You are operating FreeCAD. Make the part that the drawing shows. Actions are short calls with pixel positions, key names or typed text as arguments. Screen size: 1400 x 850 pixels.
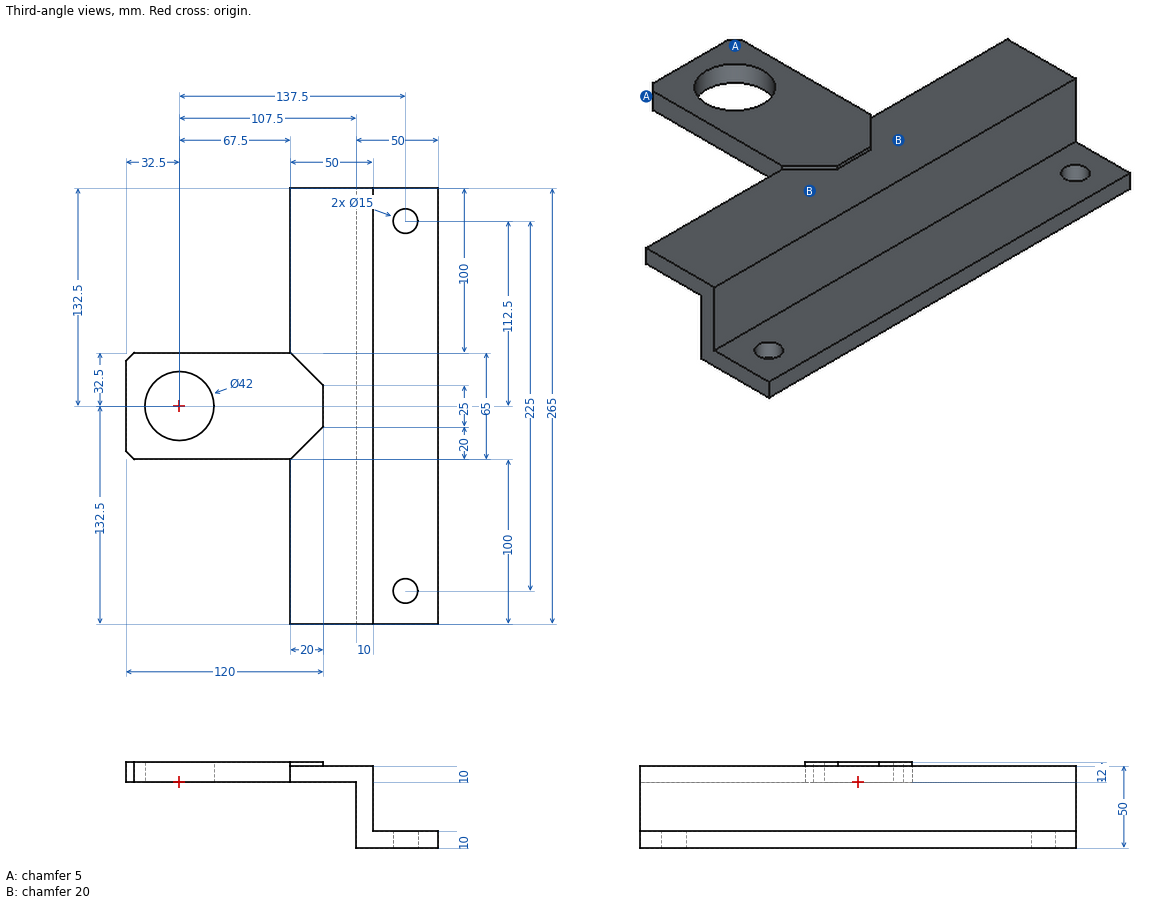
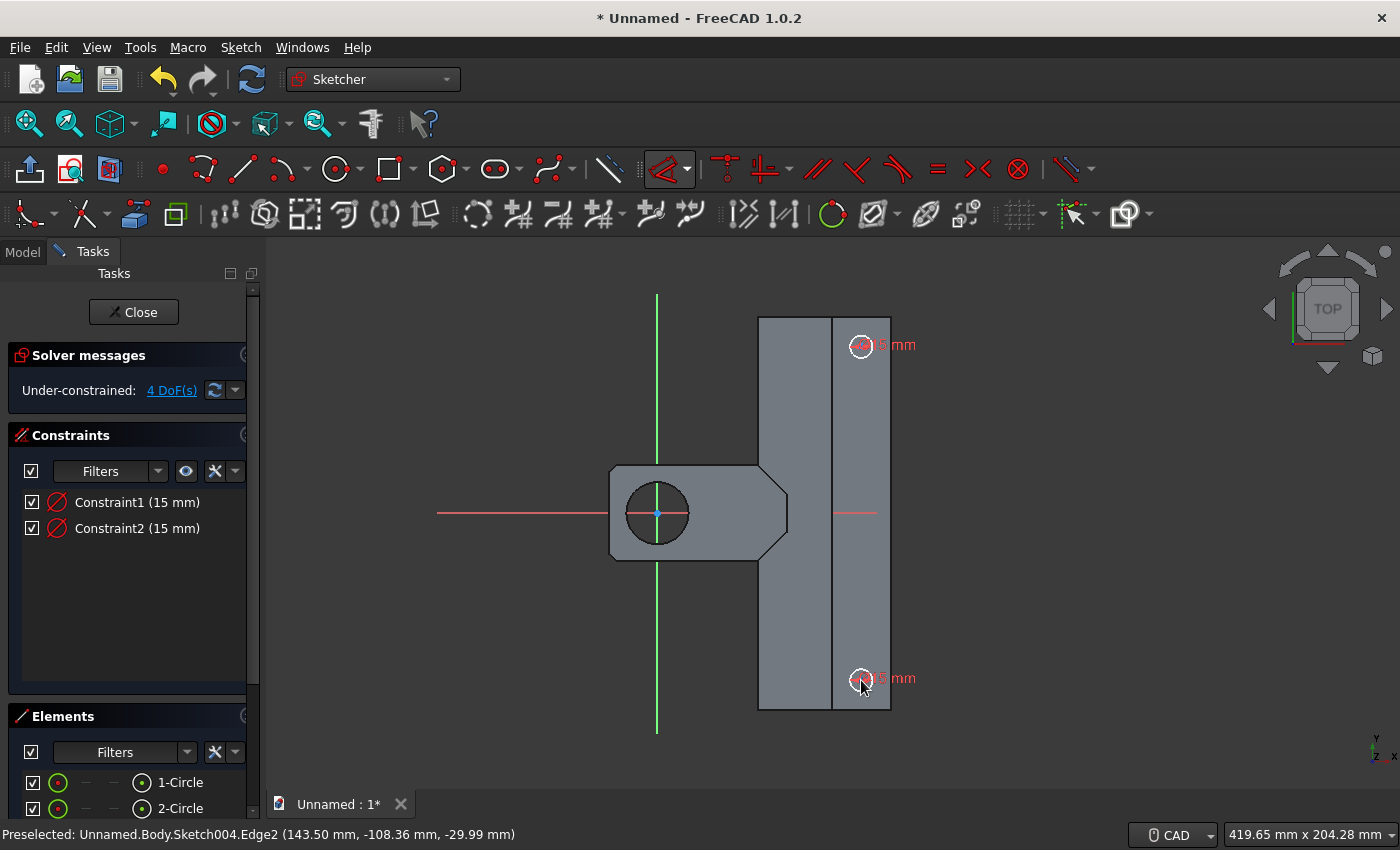
click(861, 347)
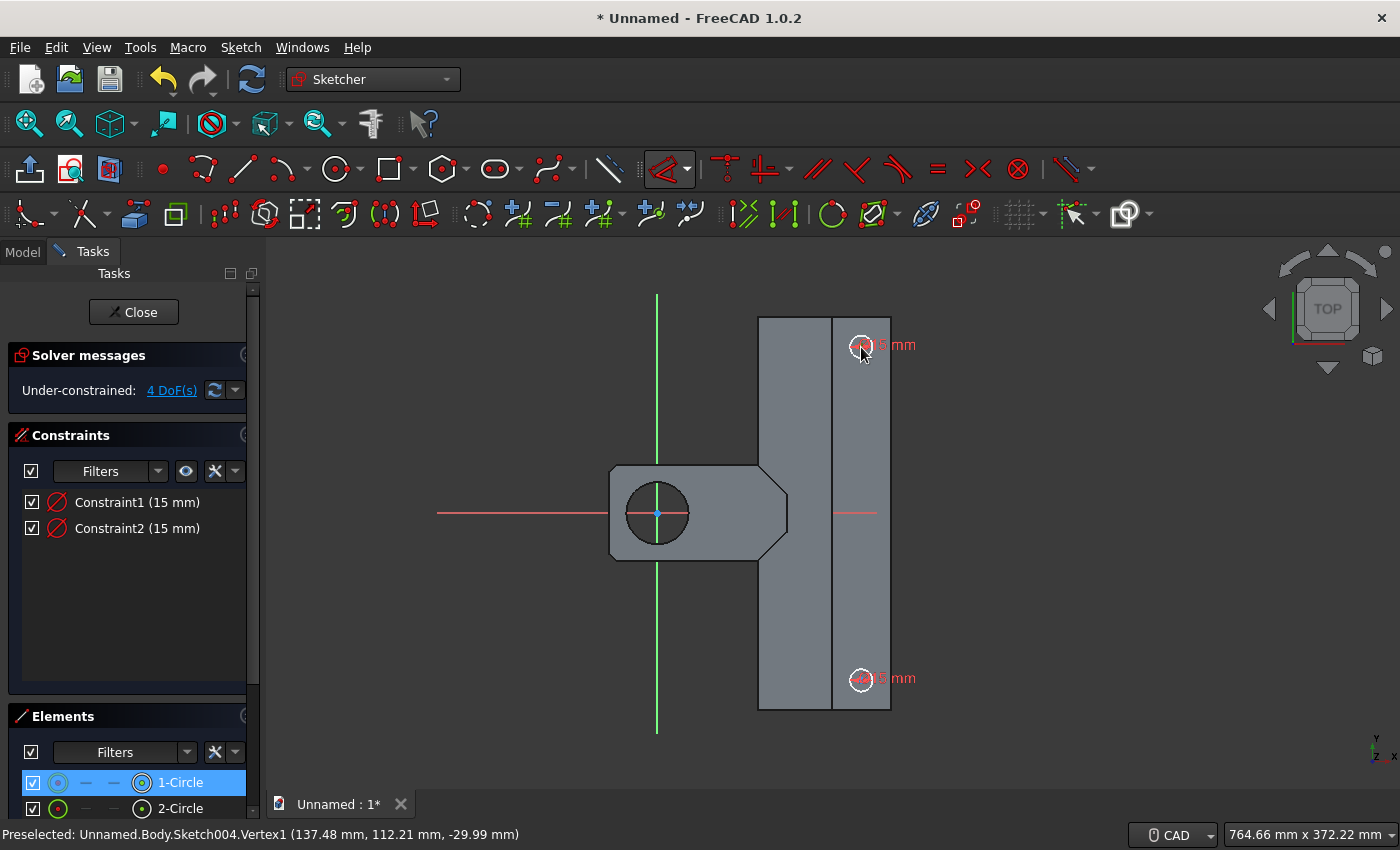
click(861, 680)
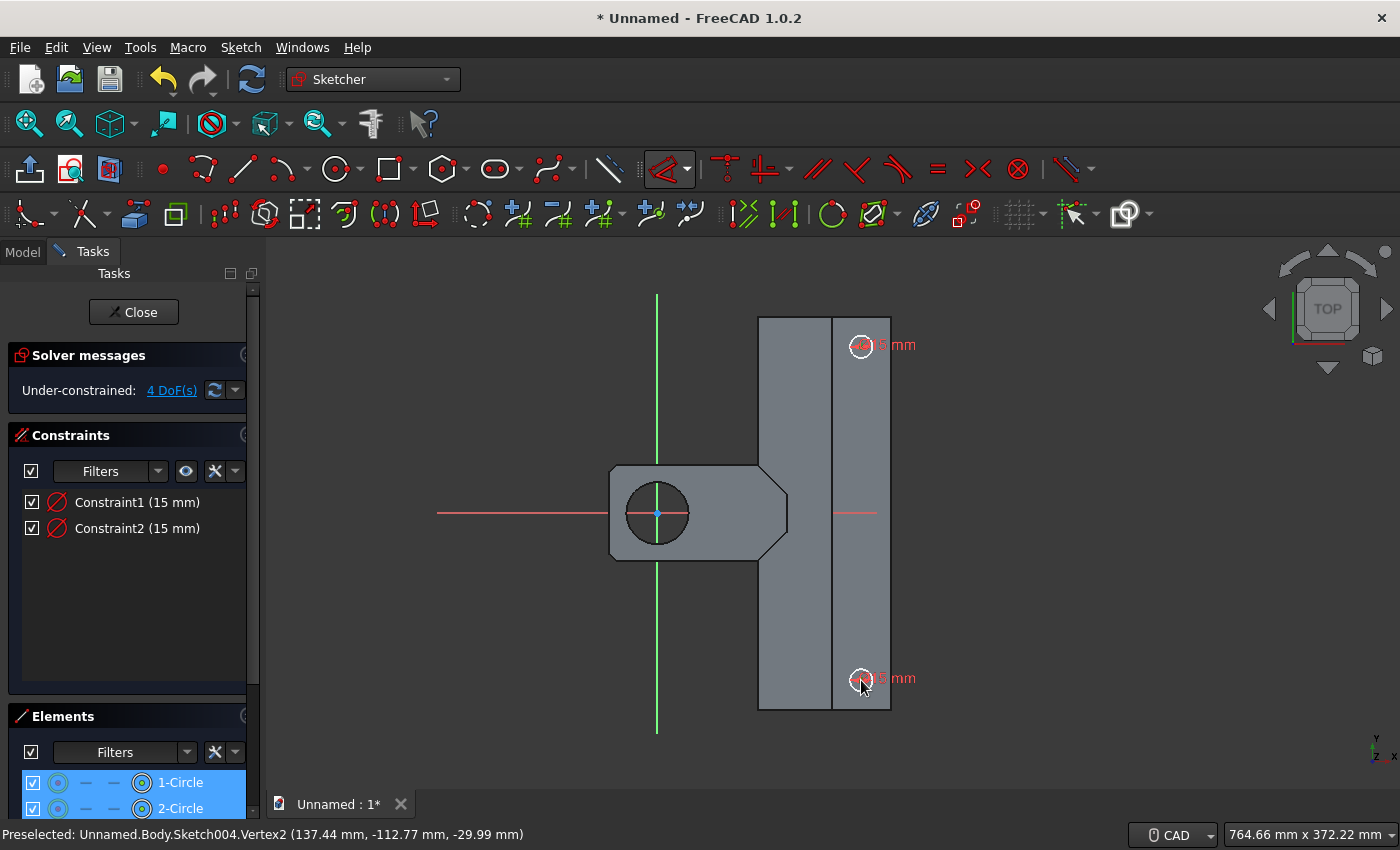
click(792, 170)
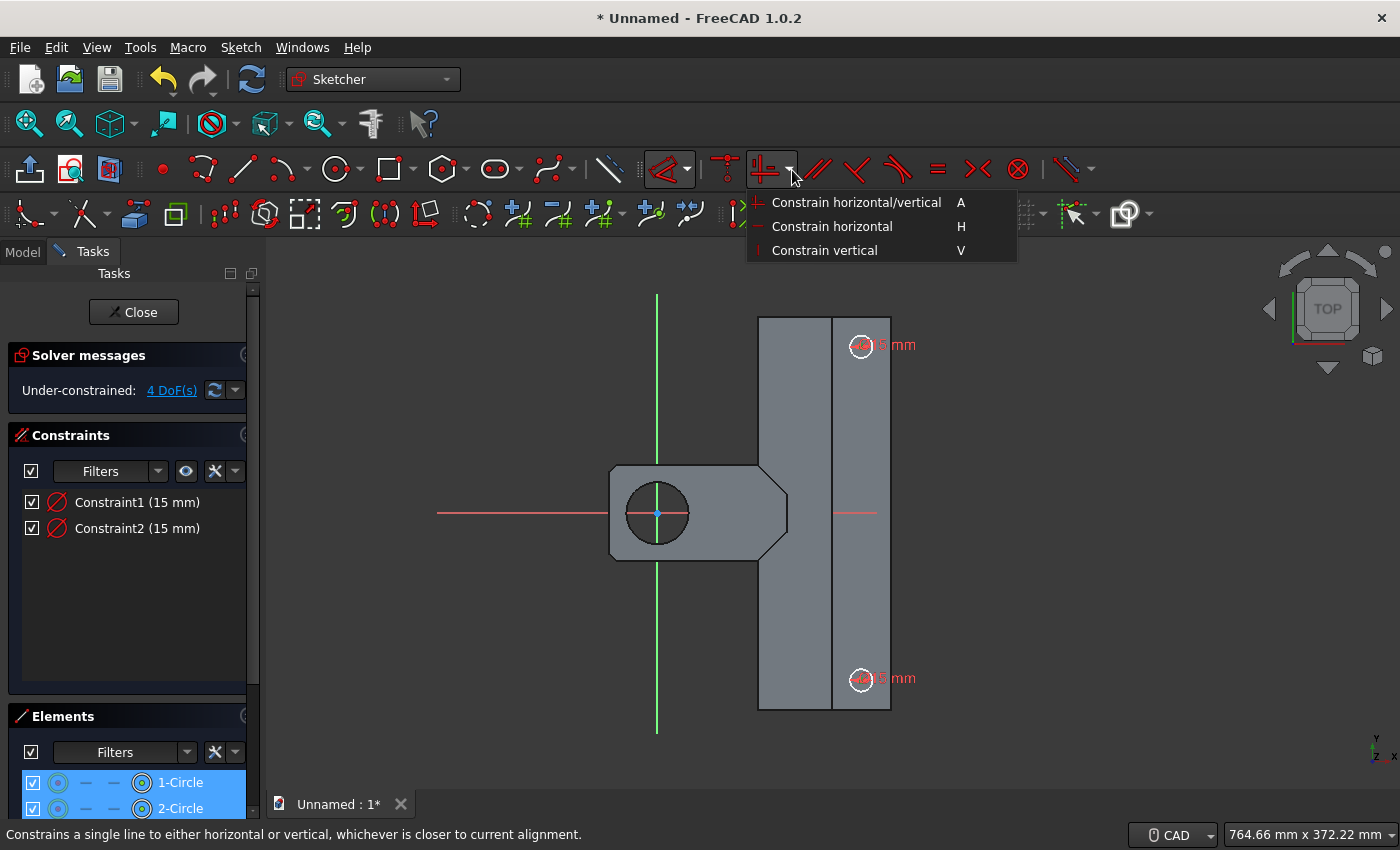
click(882, 250)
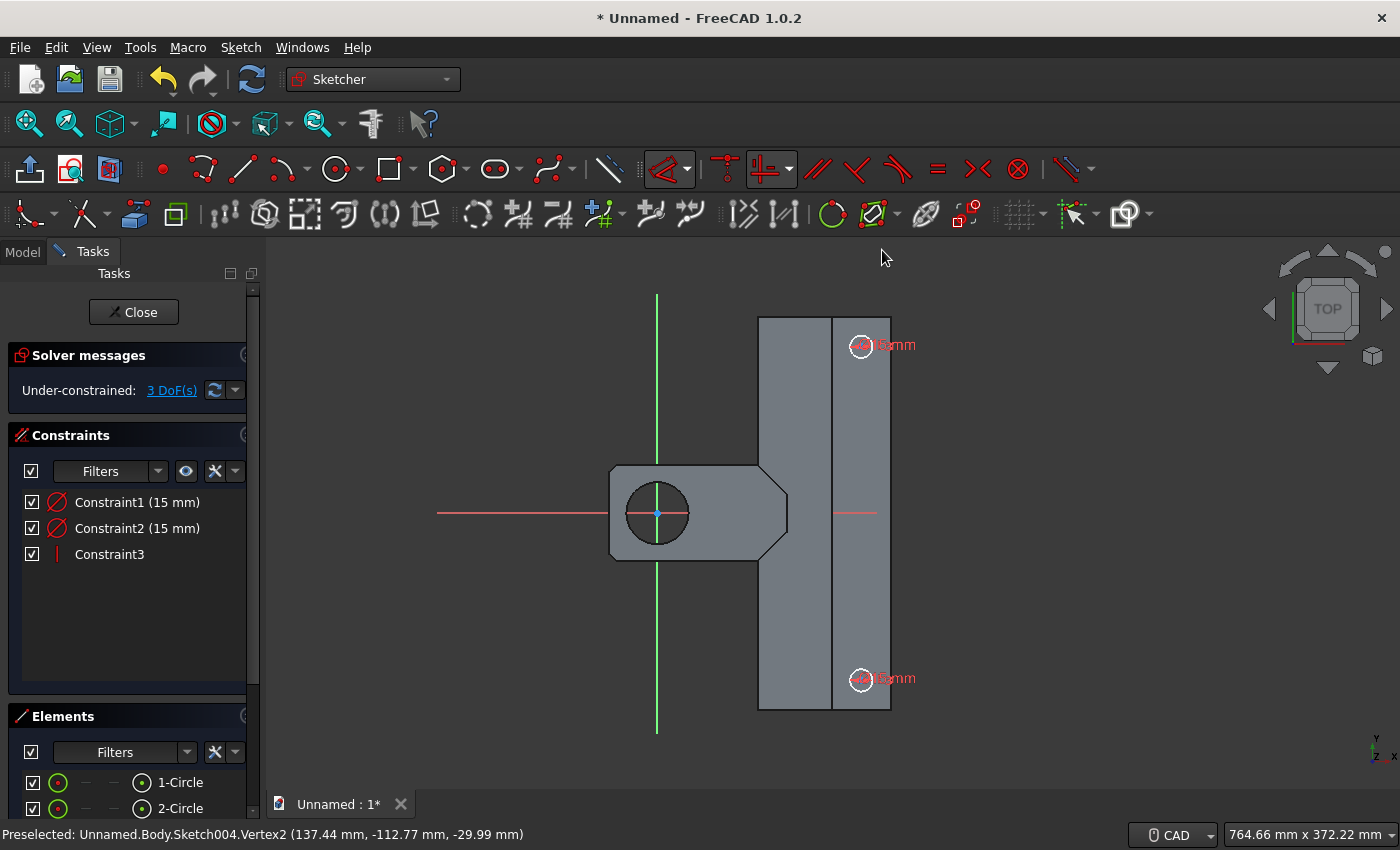
click(861, 347)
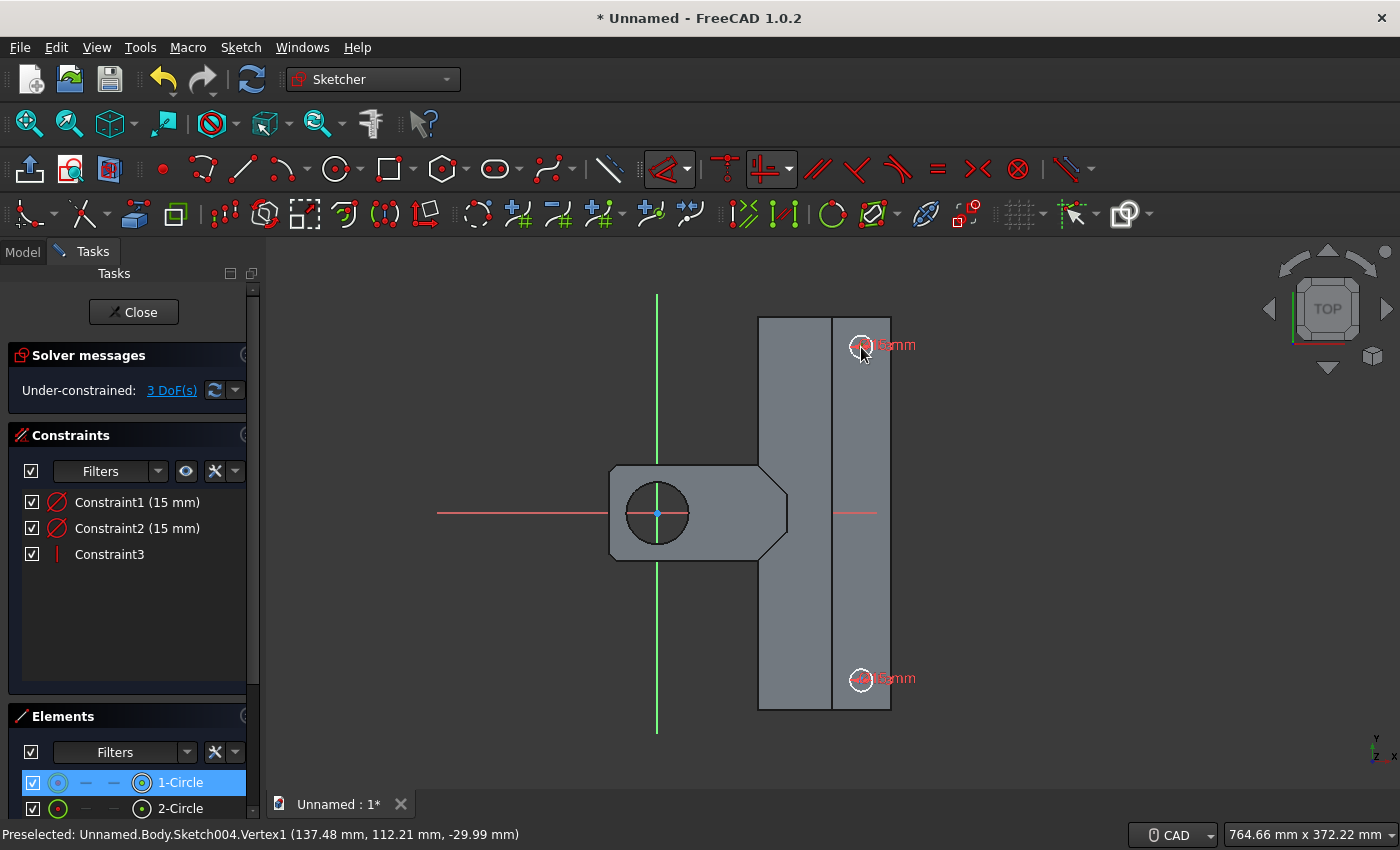
click(861, 680)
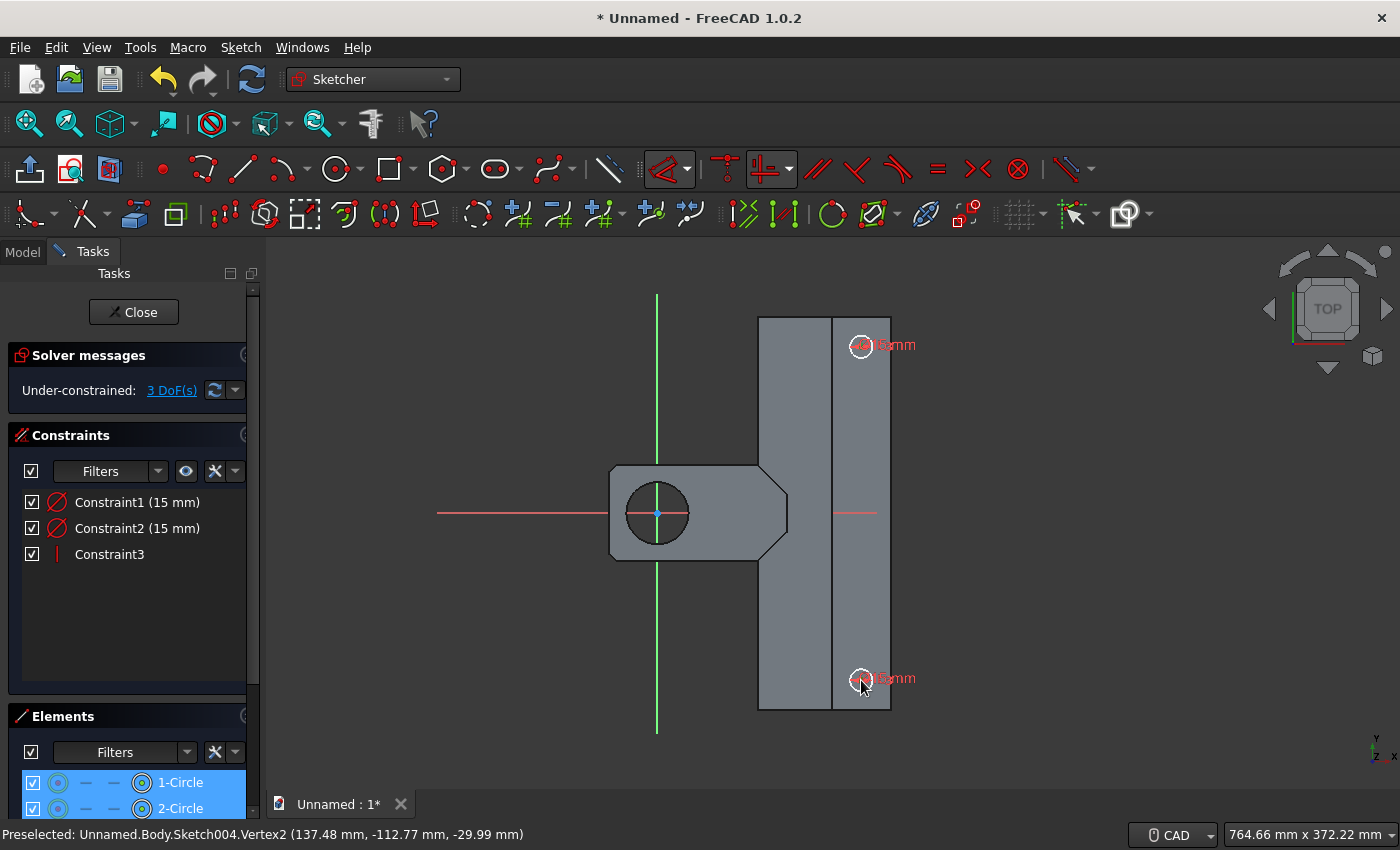
key(i)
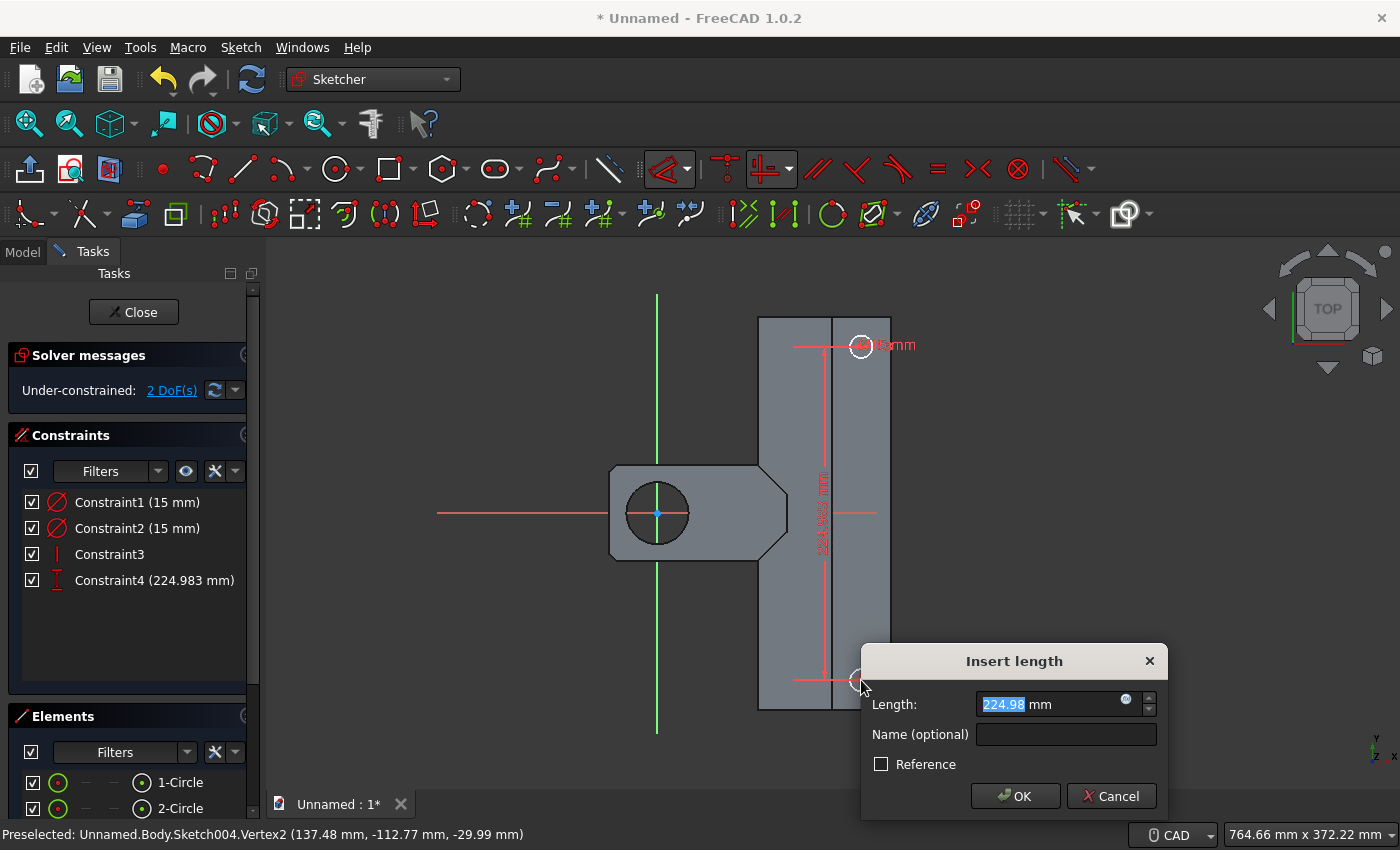
text(225)
key(Return)